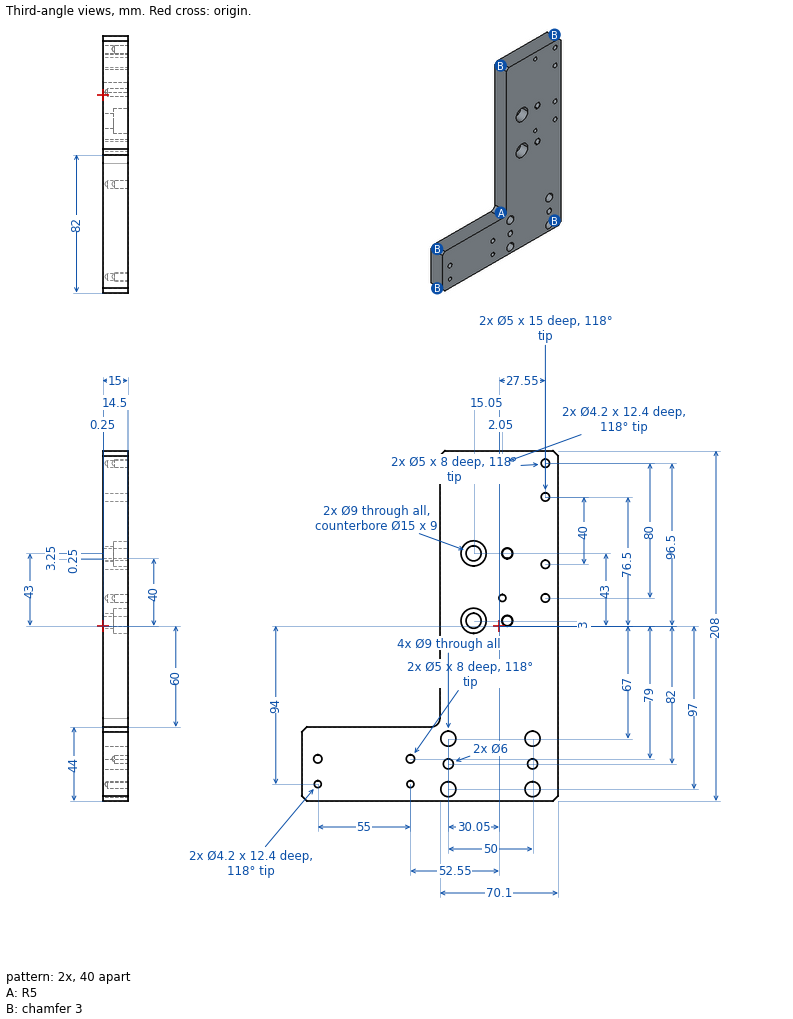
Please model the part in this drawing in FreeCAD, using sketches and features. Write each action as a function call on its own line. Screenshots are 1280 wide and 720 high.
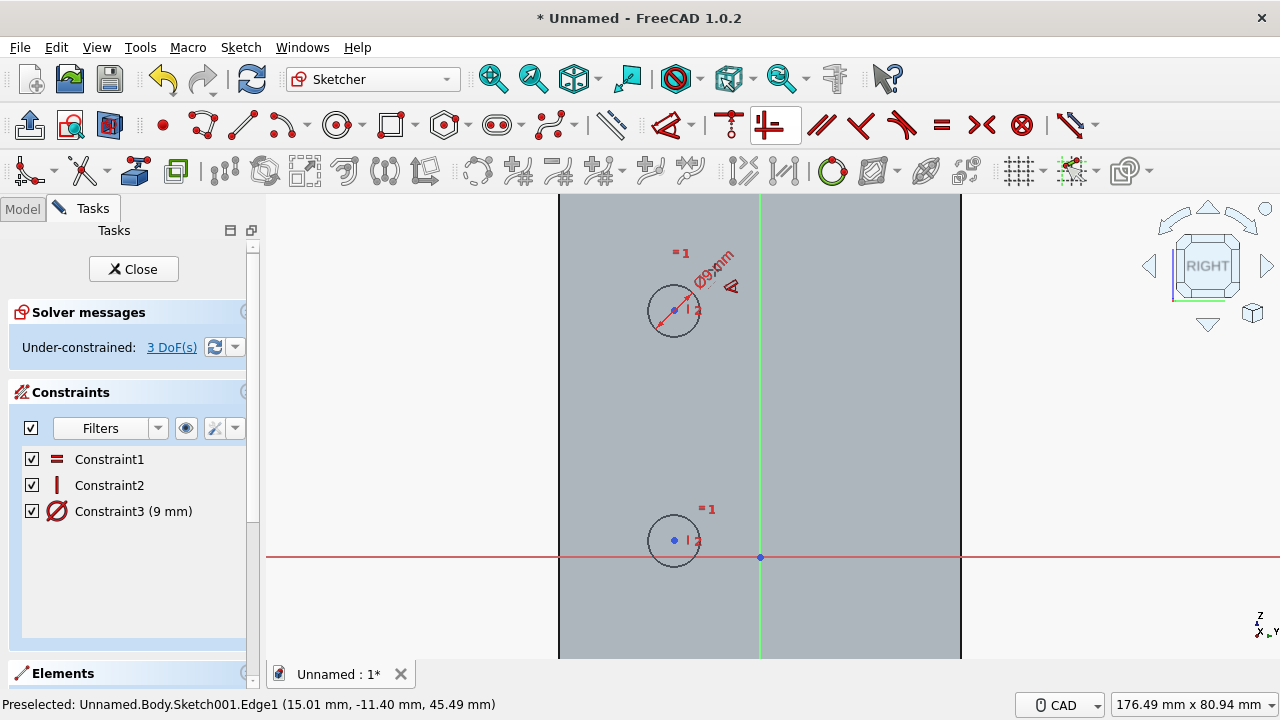
scroll(674, 541, up, 5)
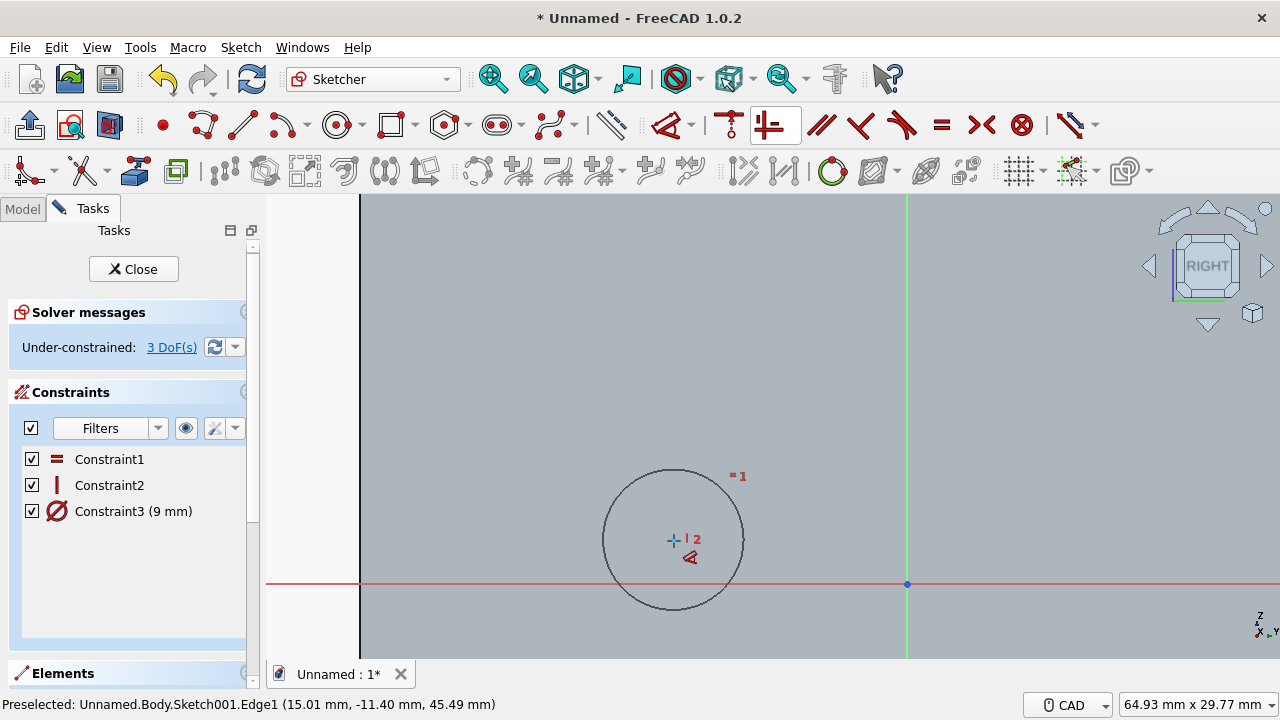
click(673, 540)
click(941, 562)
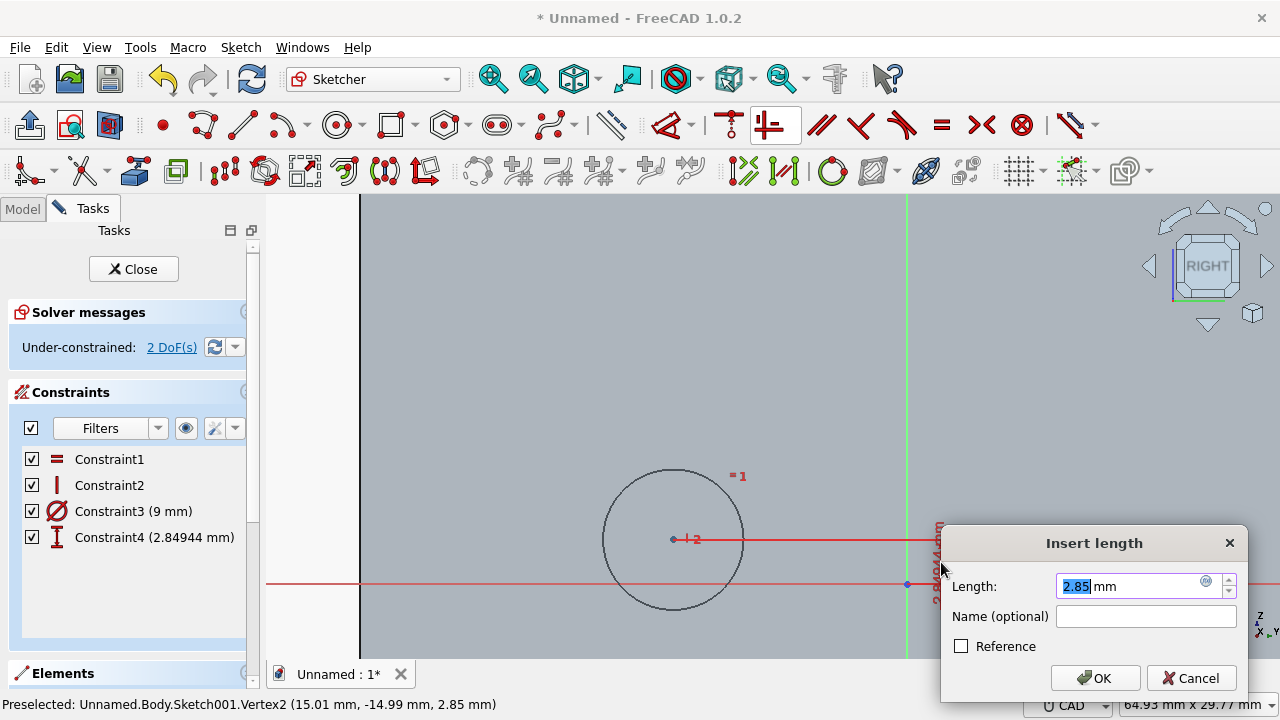
text(3)
key(Return)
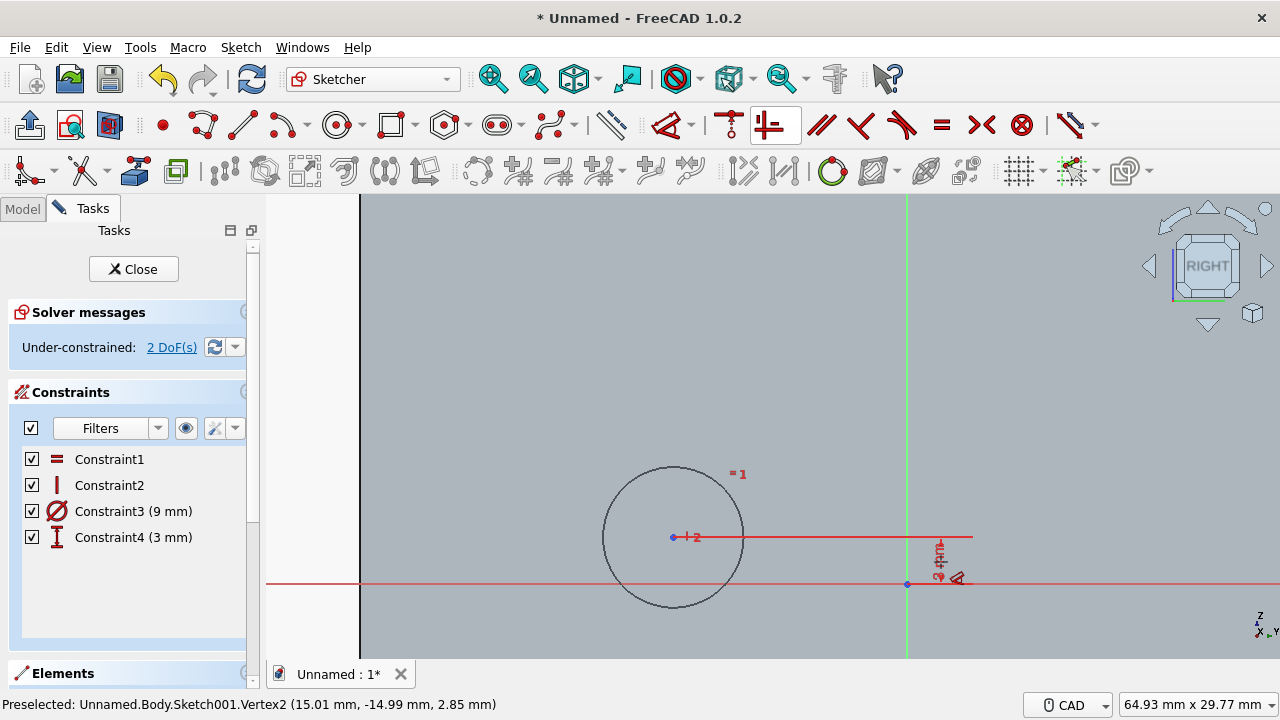
scroll(675, 544, down, 5)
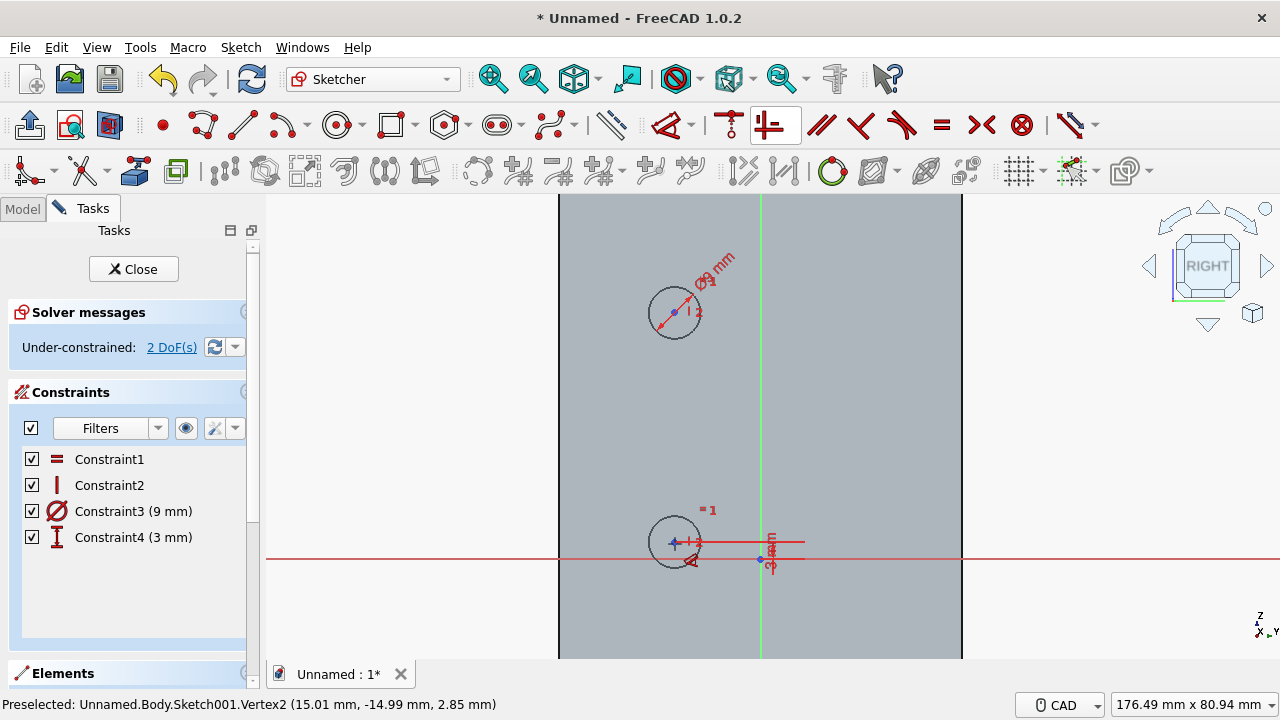
click(675, 313)
click(795, 436)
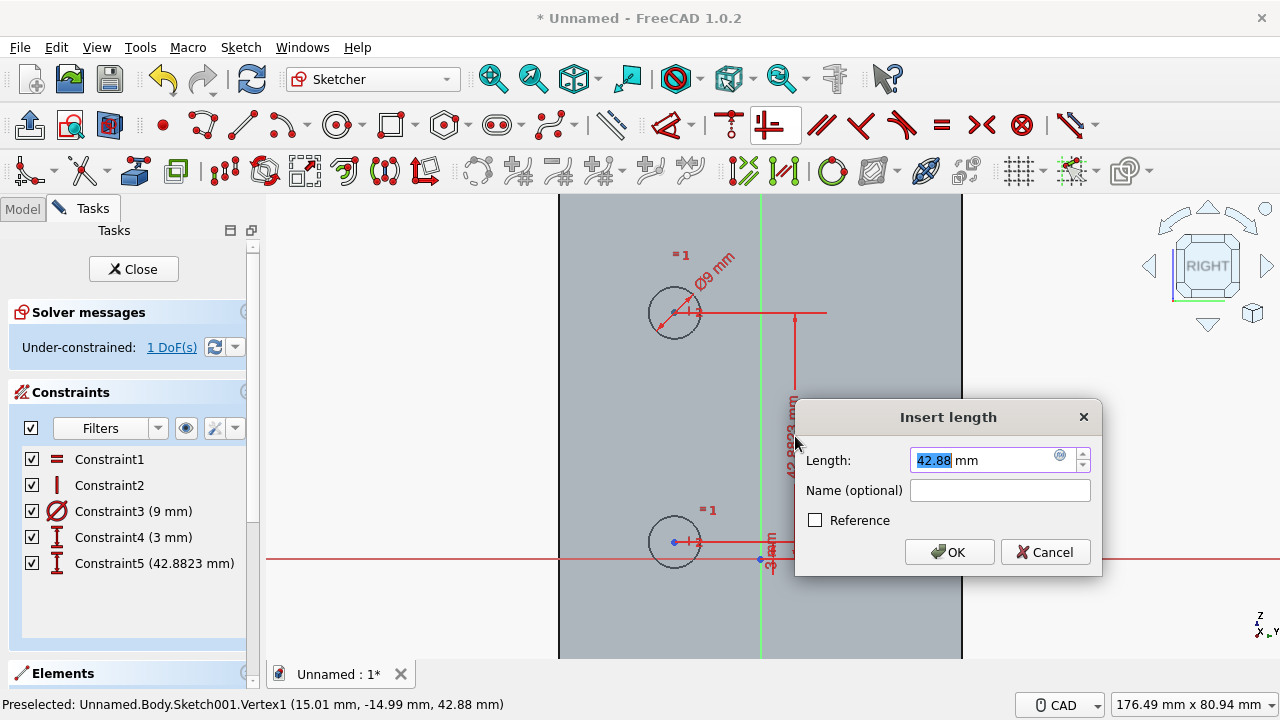
text(43)
key(Return)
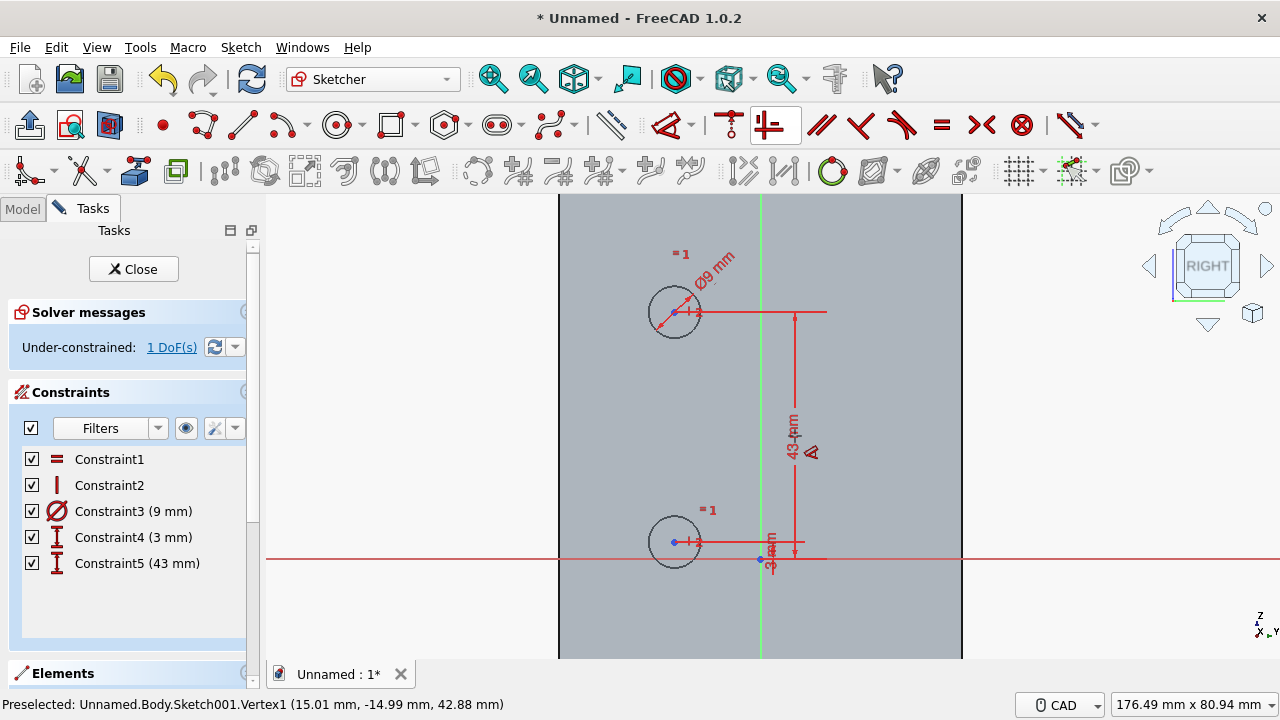
click(675, 312)
click(718, 593)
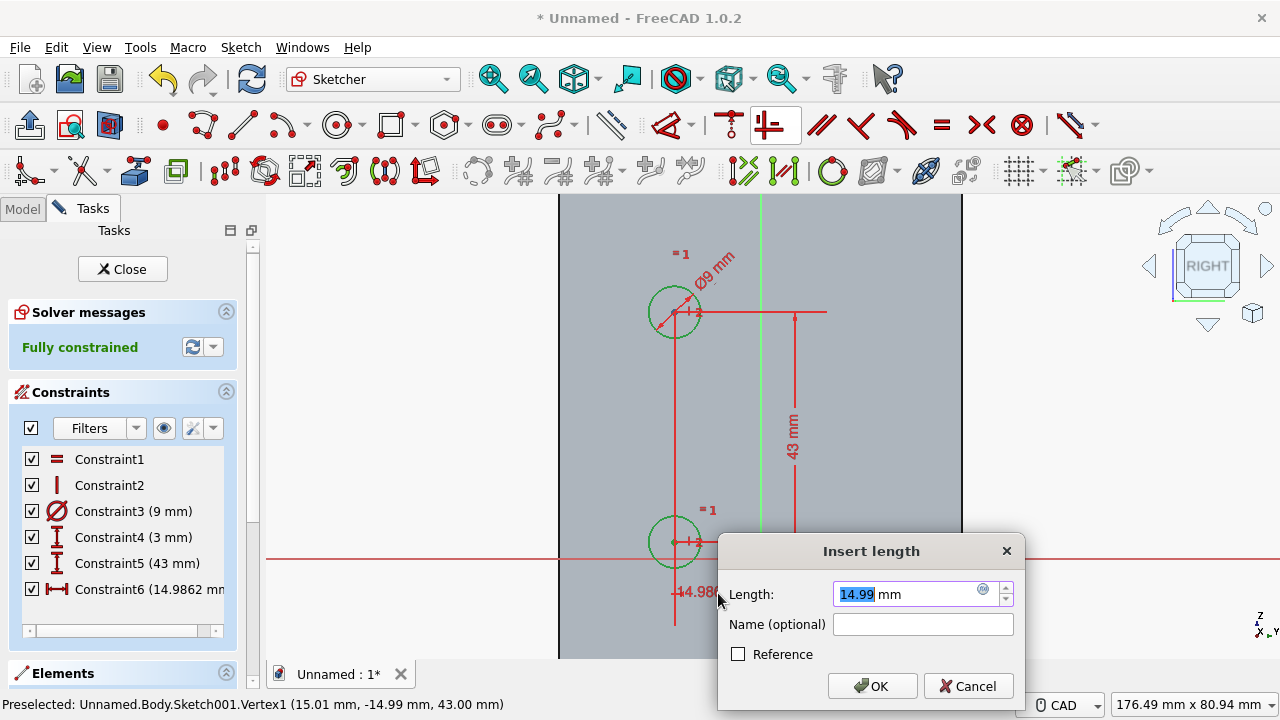
text(15.05)
key(Return)
key(Escape)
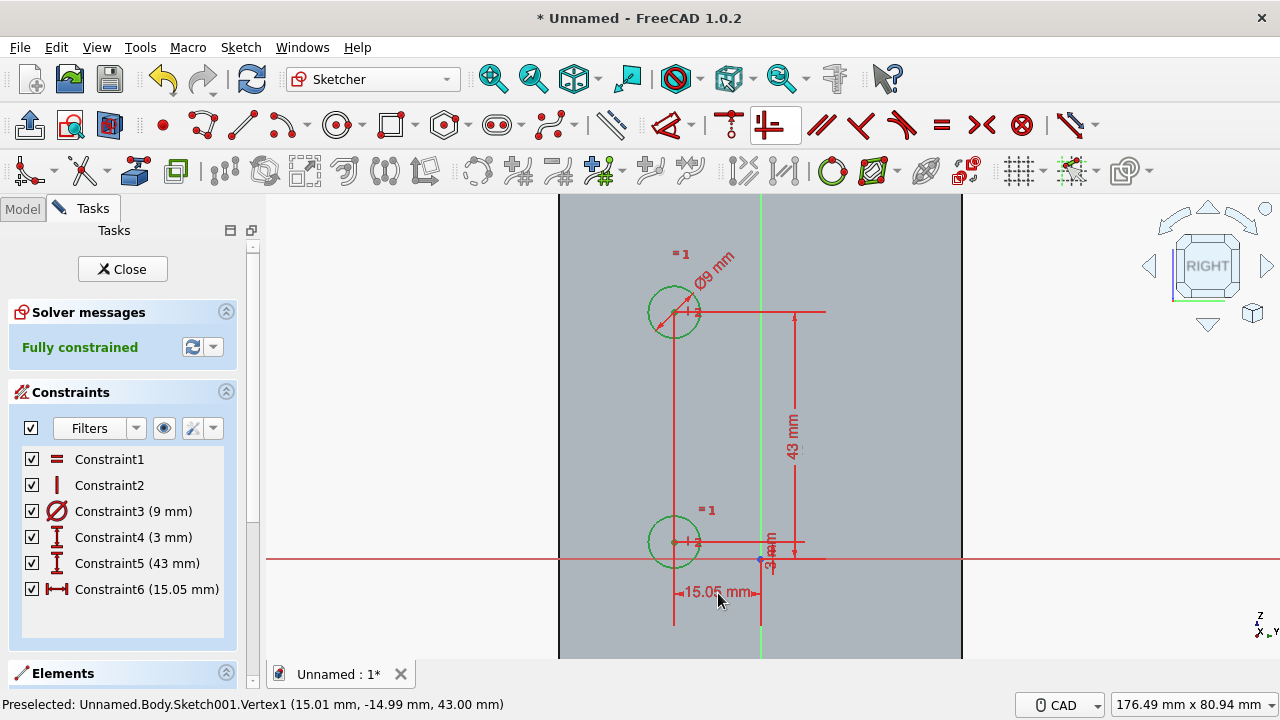
click(123, 269)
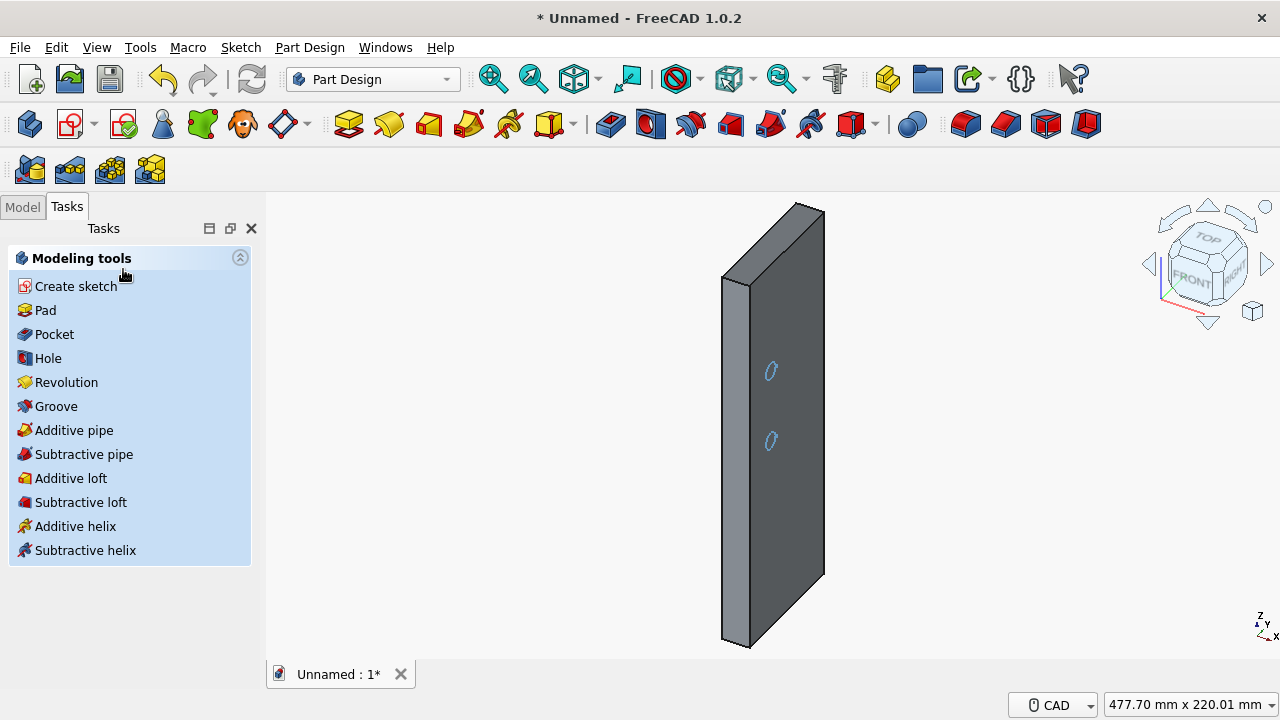
click(652, 124)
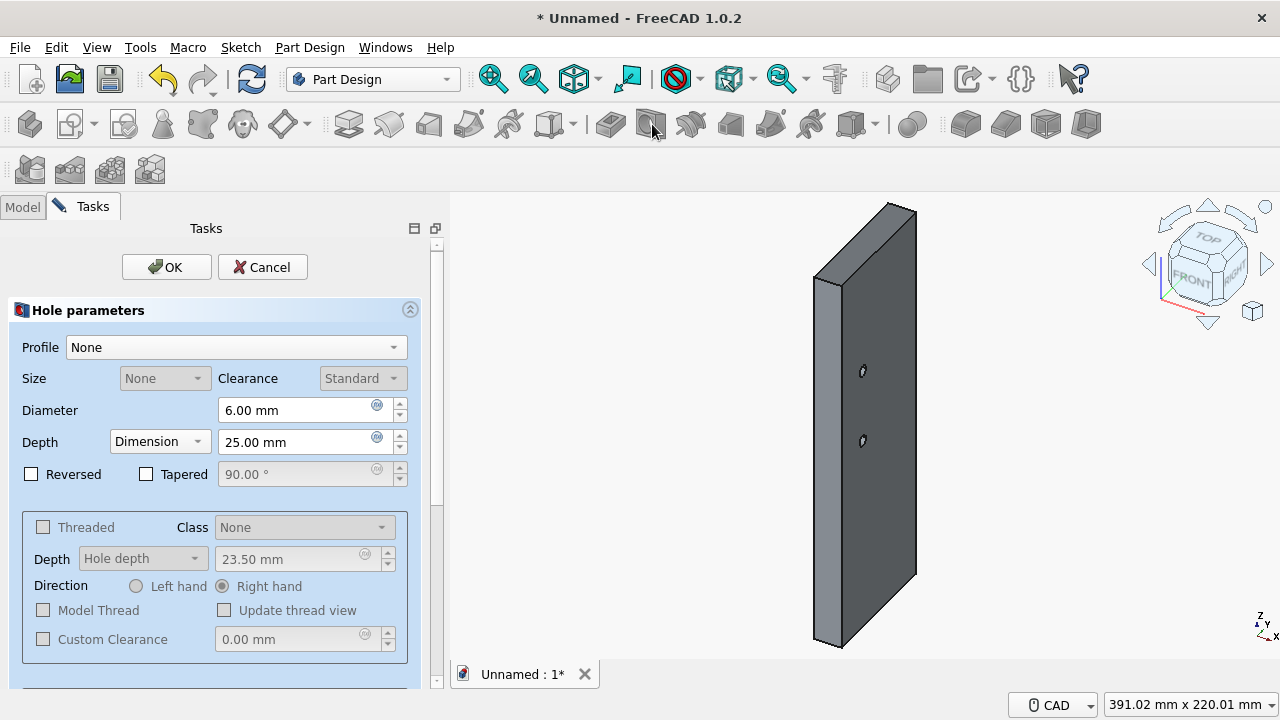
triple_click(305, 410)